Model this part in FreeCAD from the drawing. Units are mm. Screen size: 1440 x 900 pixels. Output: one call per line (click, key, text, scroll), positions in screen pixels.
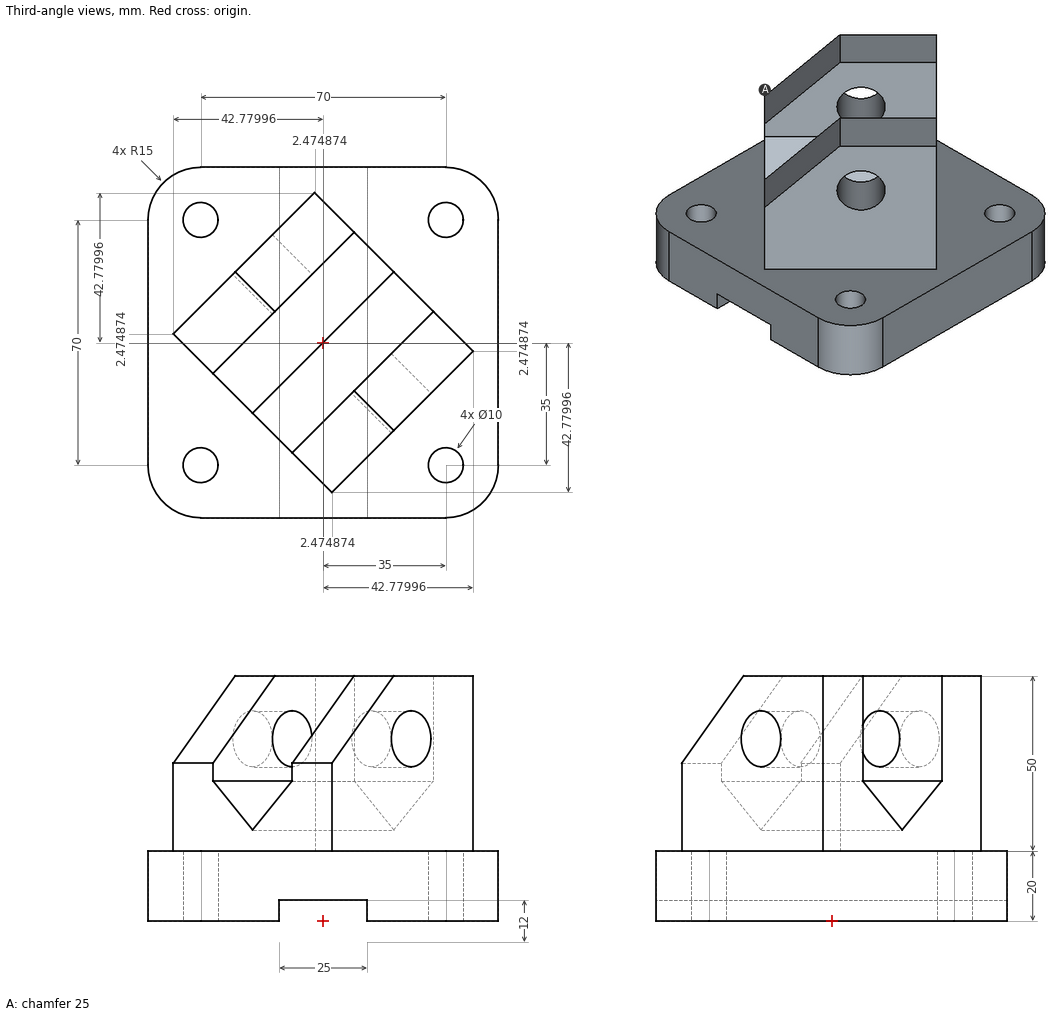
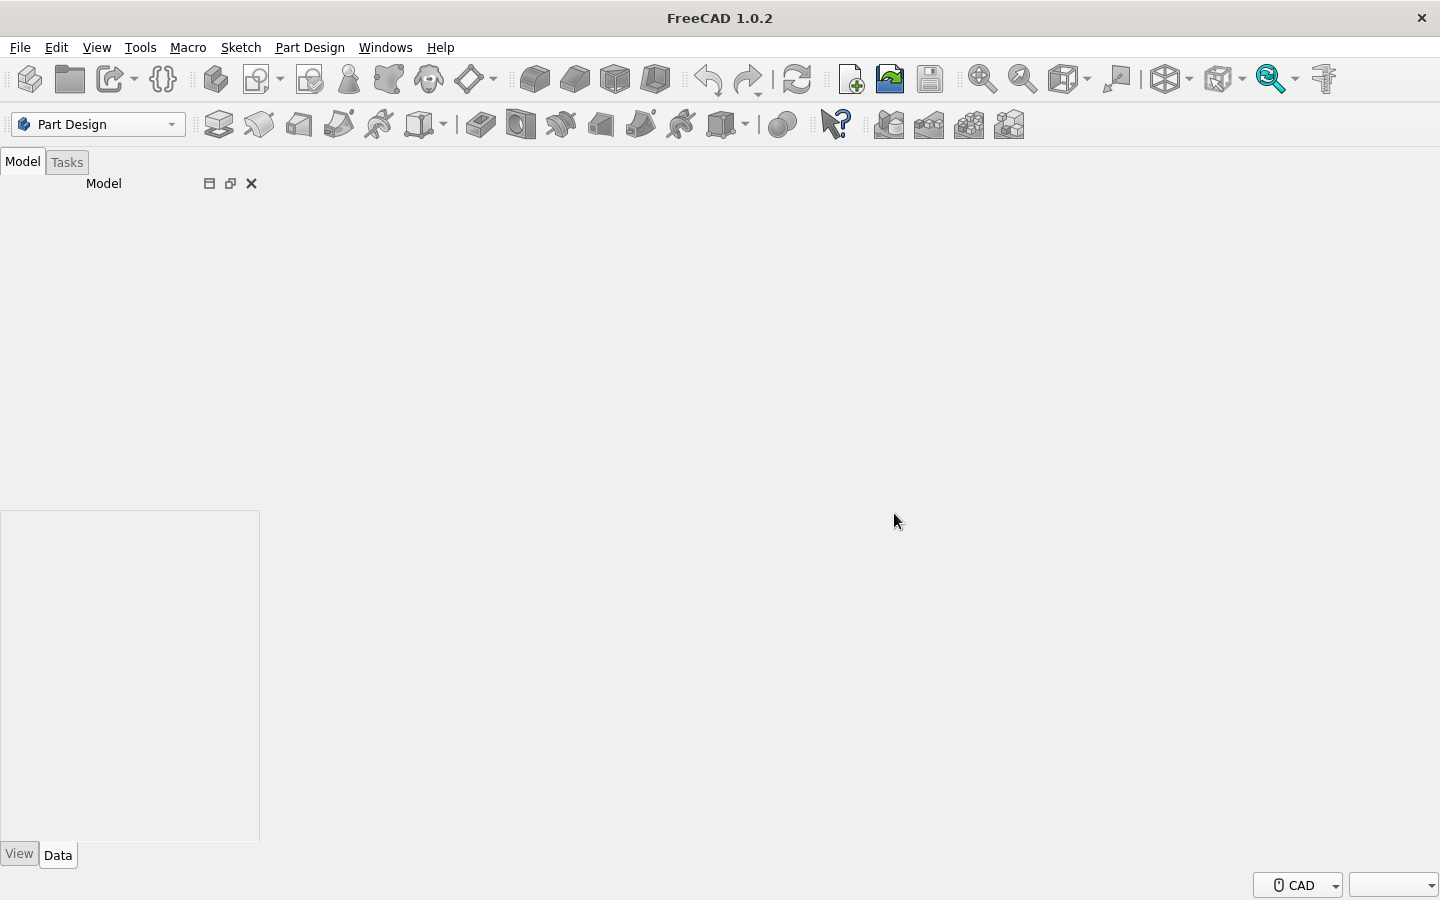
click(850, 80)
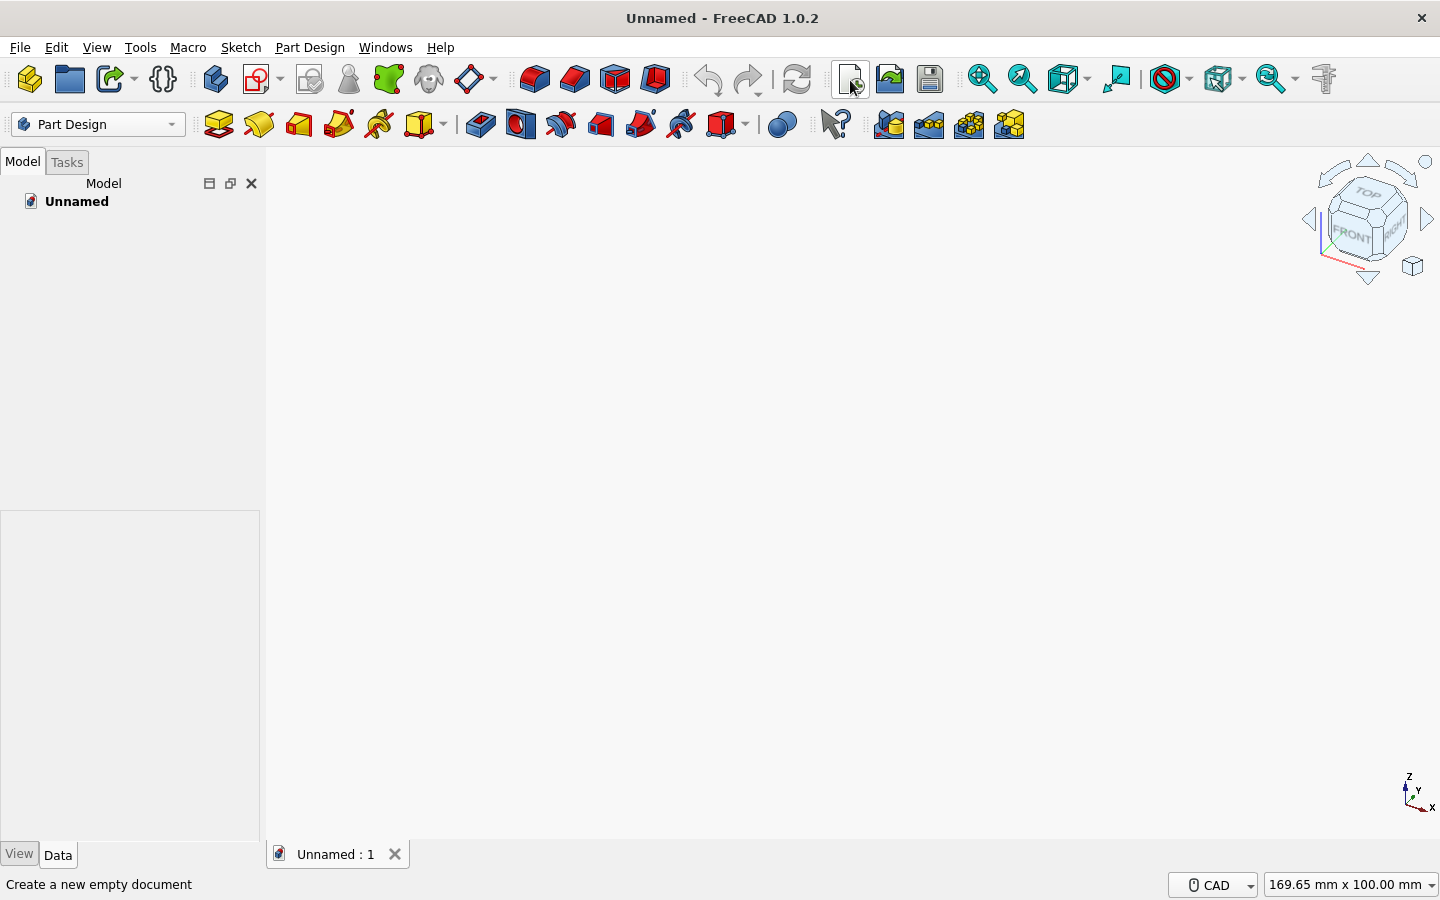
click(256, 80)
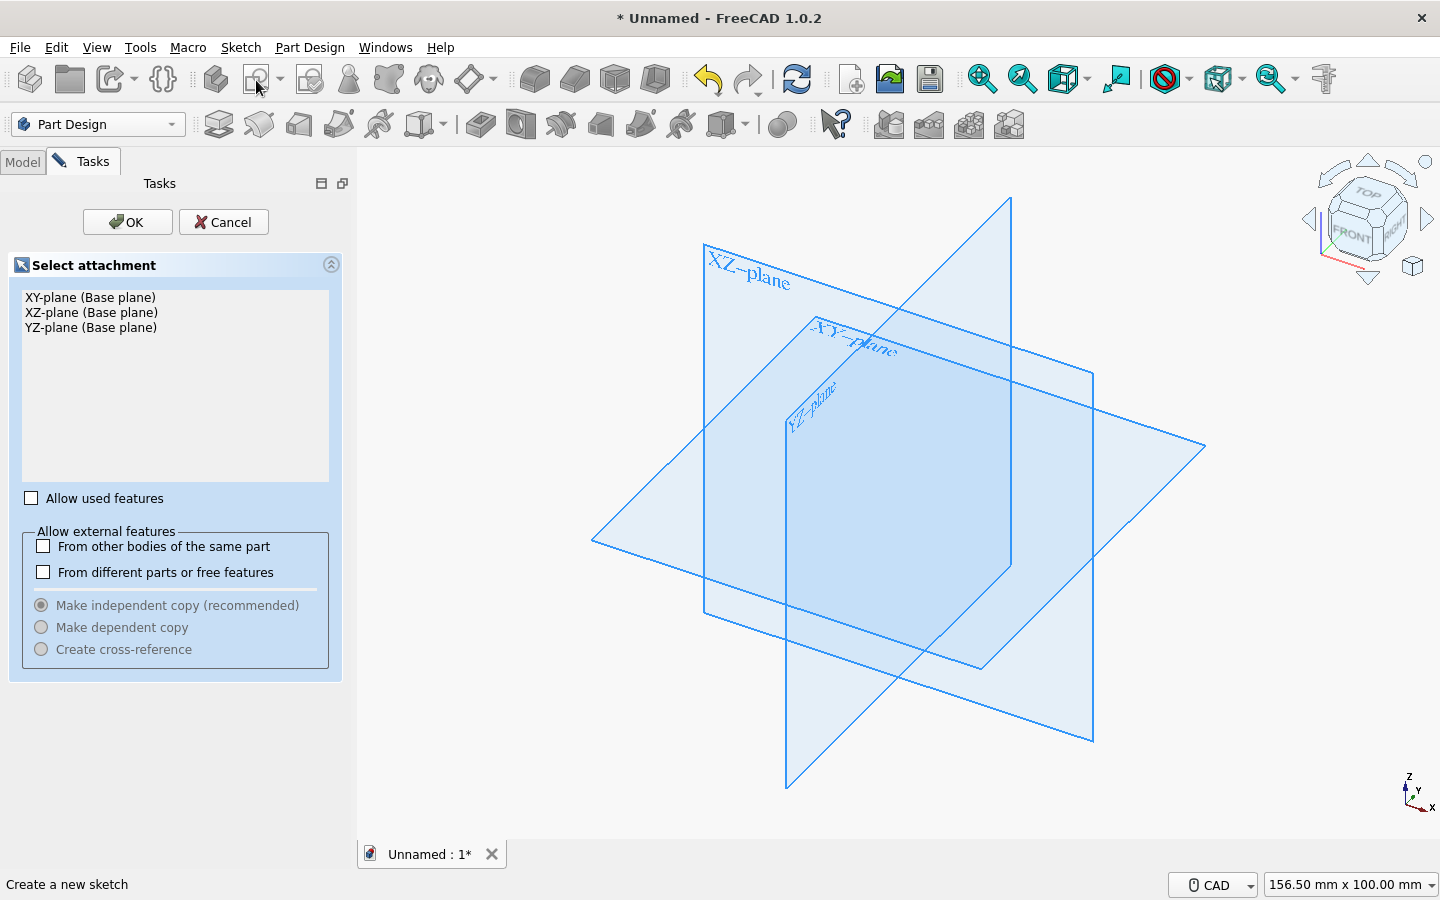
click(82, 298)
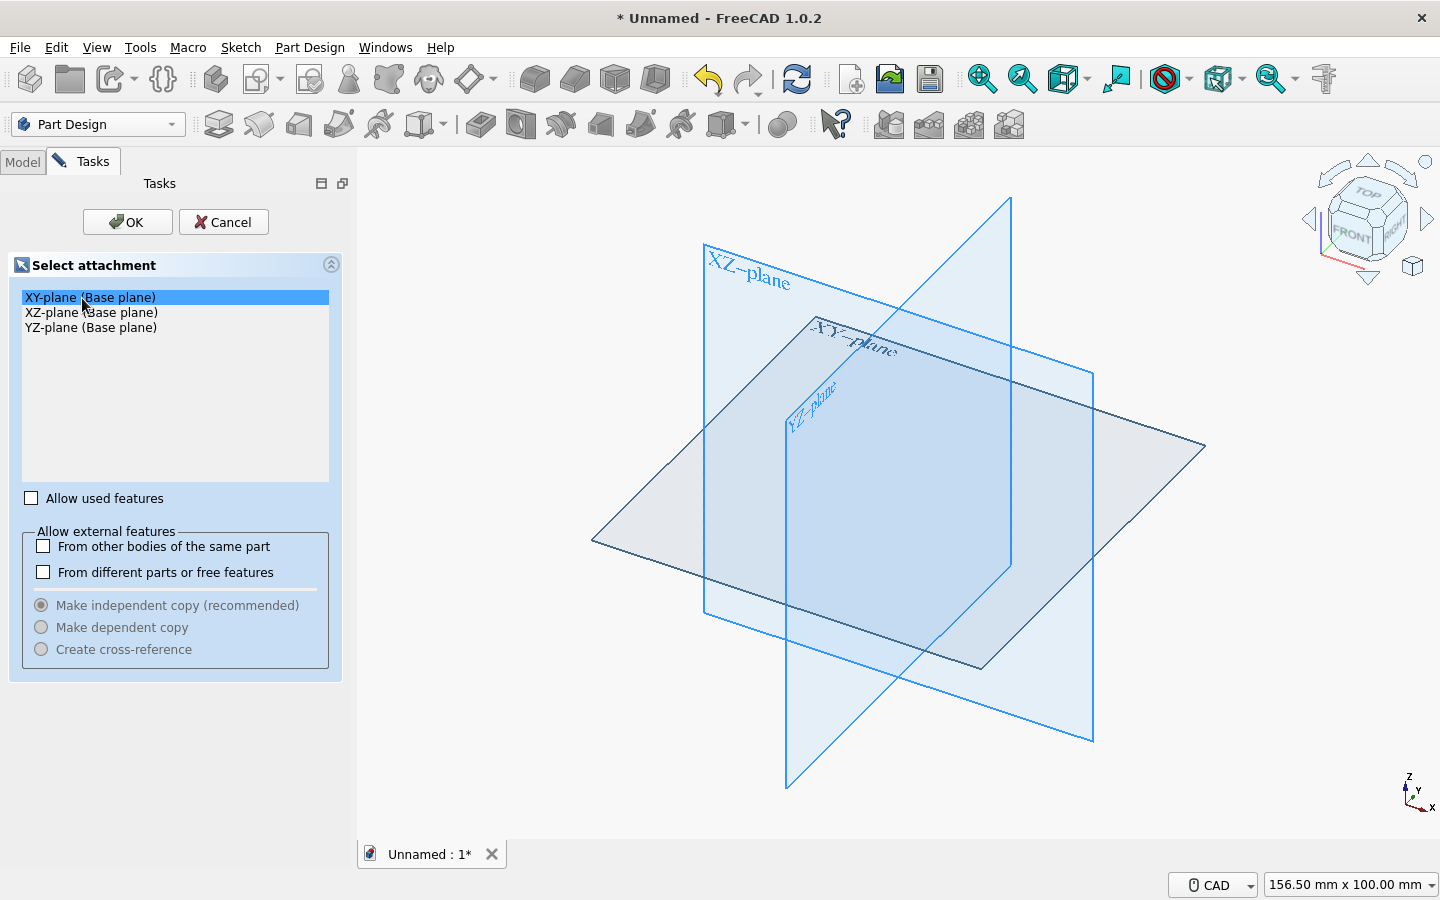
click(128, 222)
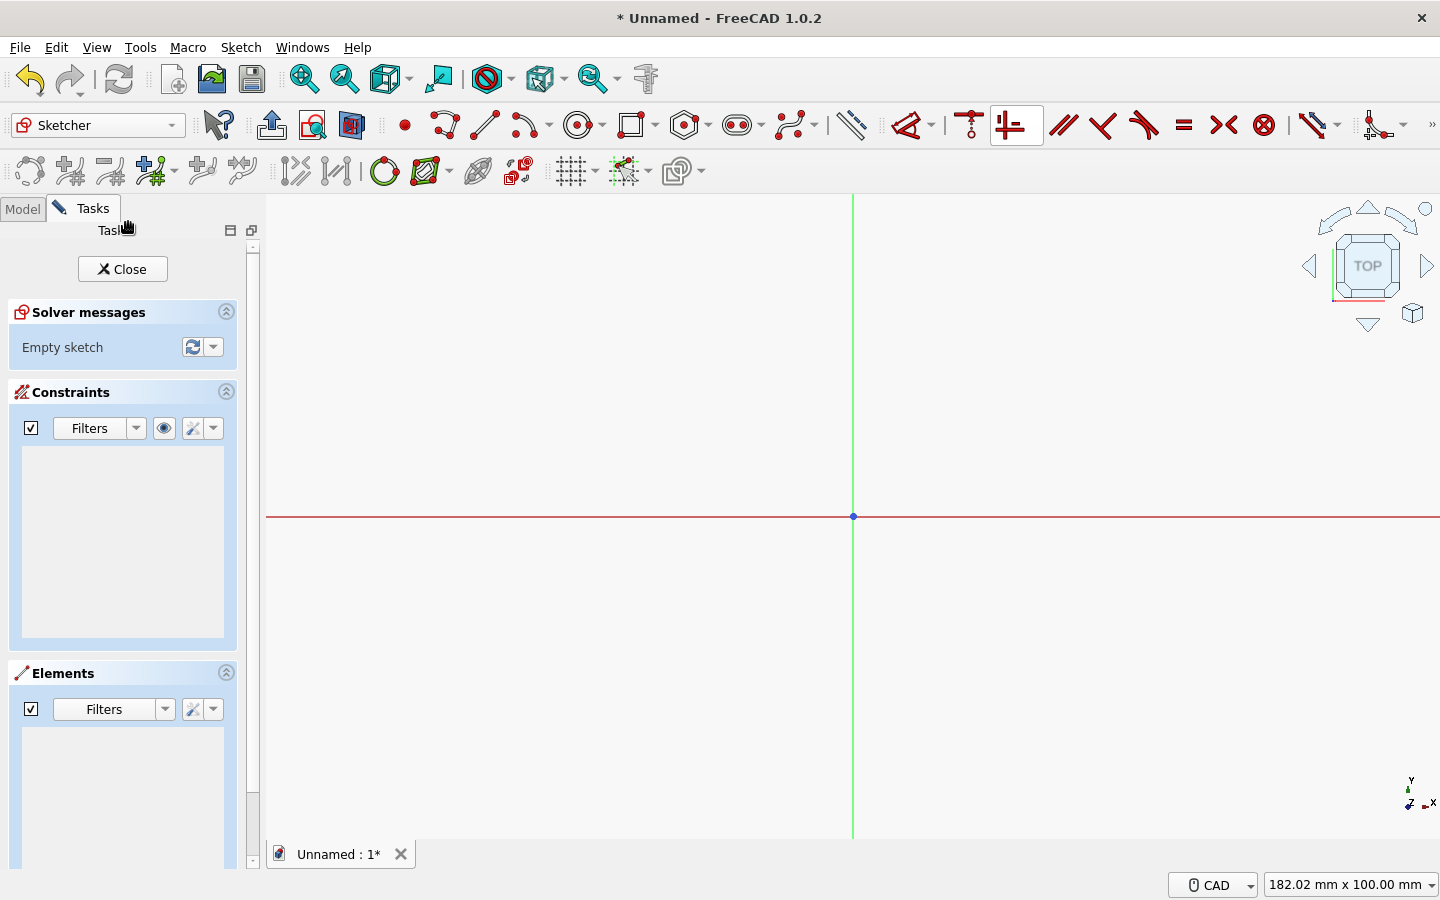
scroll(645, 516, down, 2)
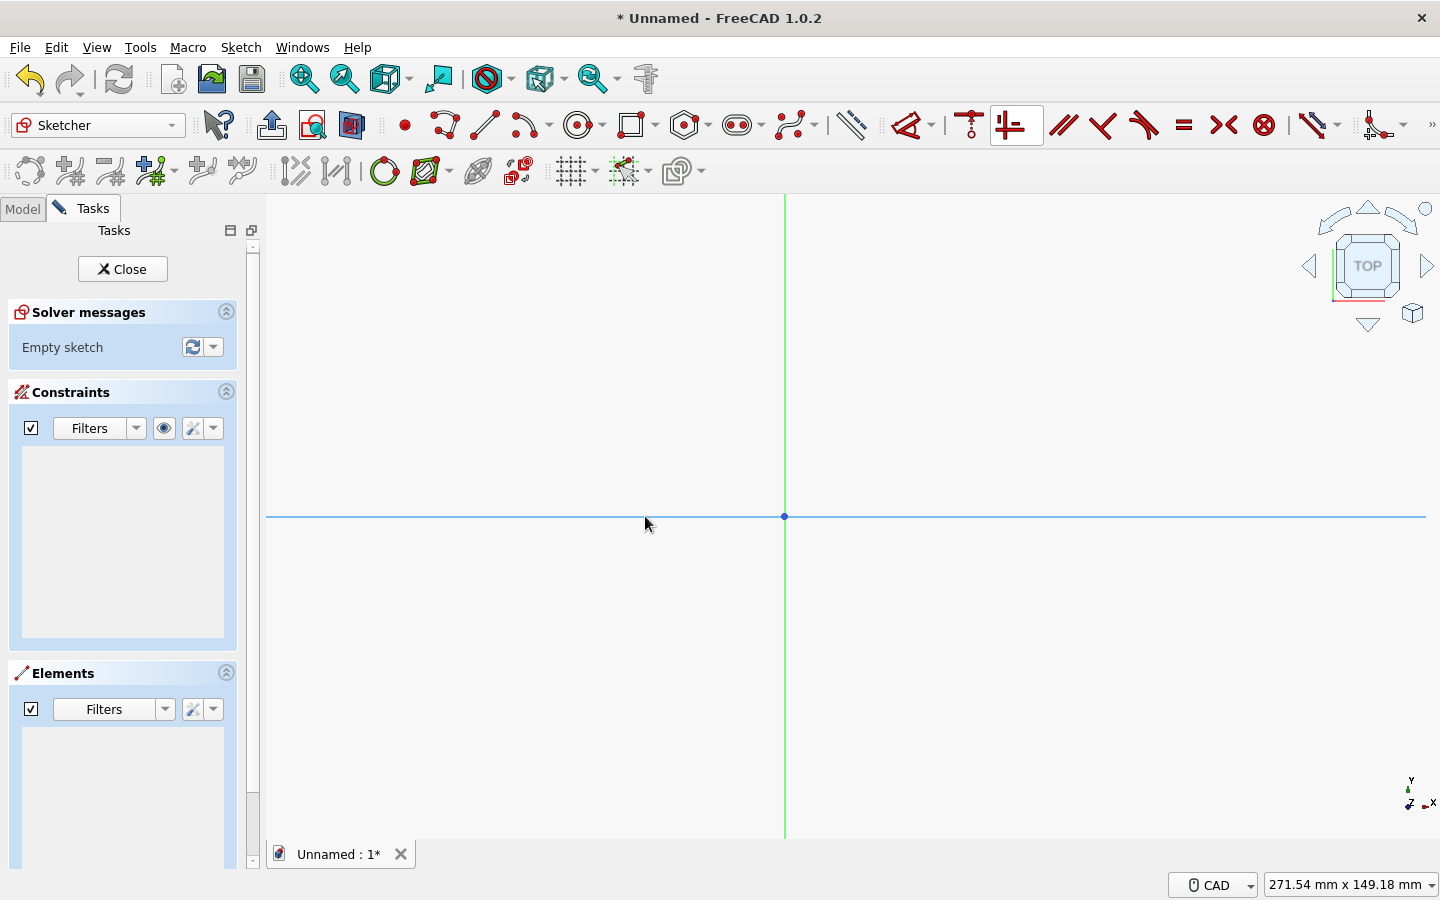
key(g)
key(l)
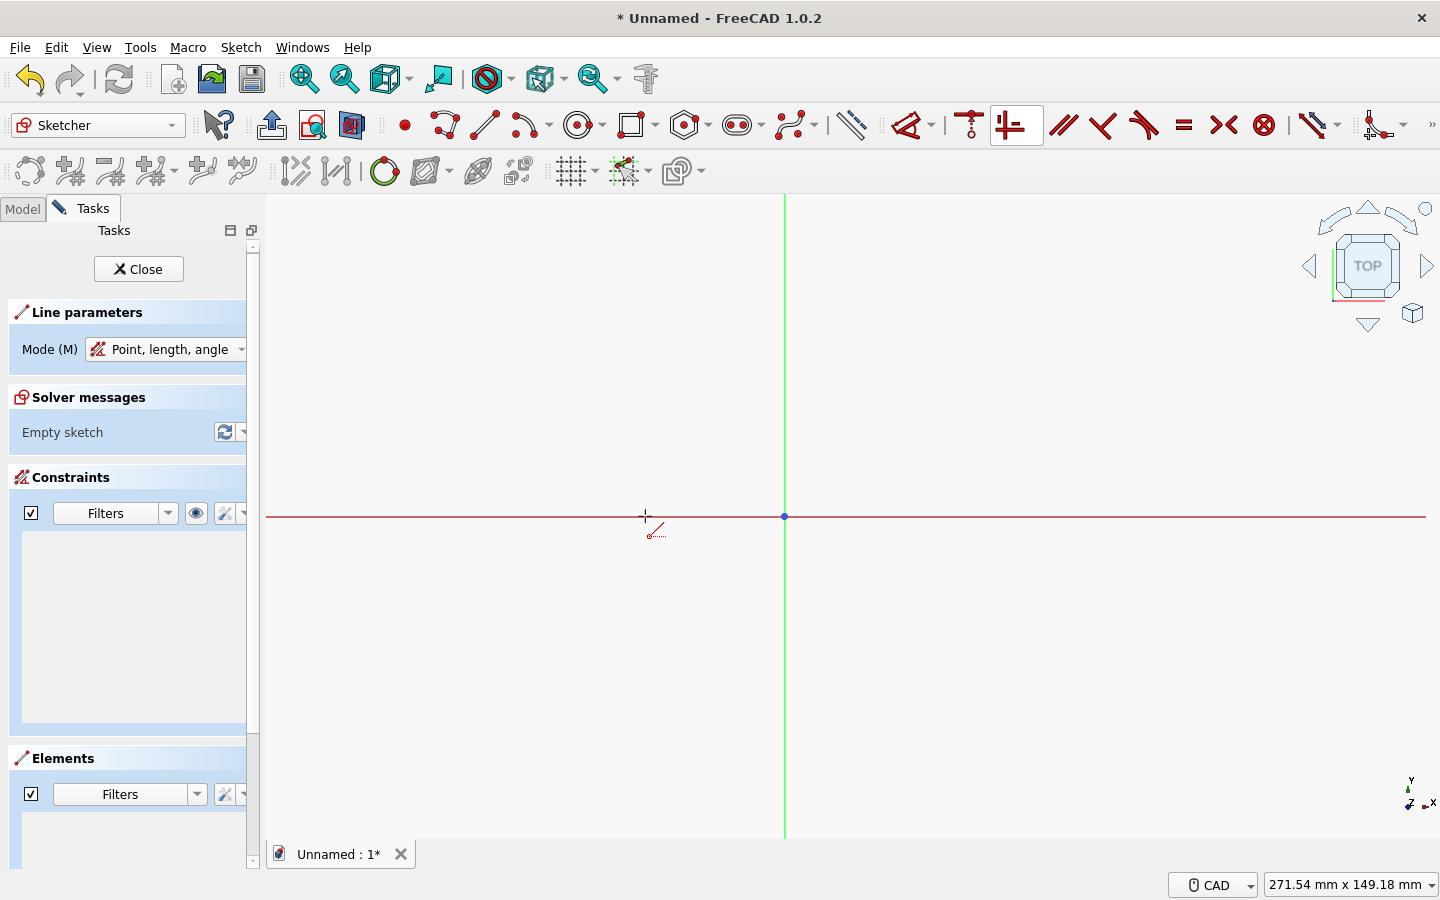
click(936, 300)
click(633, 300)